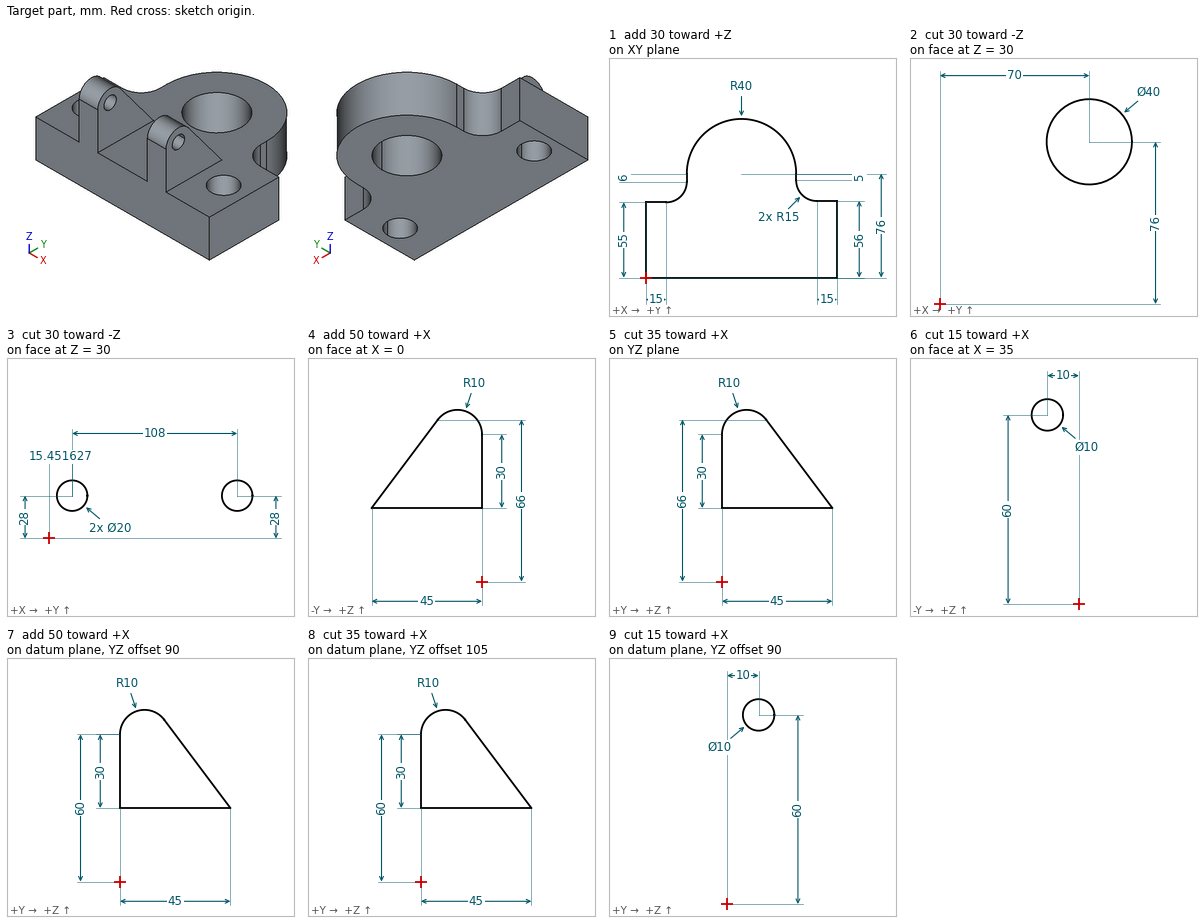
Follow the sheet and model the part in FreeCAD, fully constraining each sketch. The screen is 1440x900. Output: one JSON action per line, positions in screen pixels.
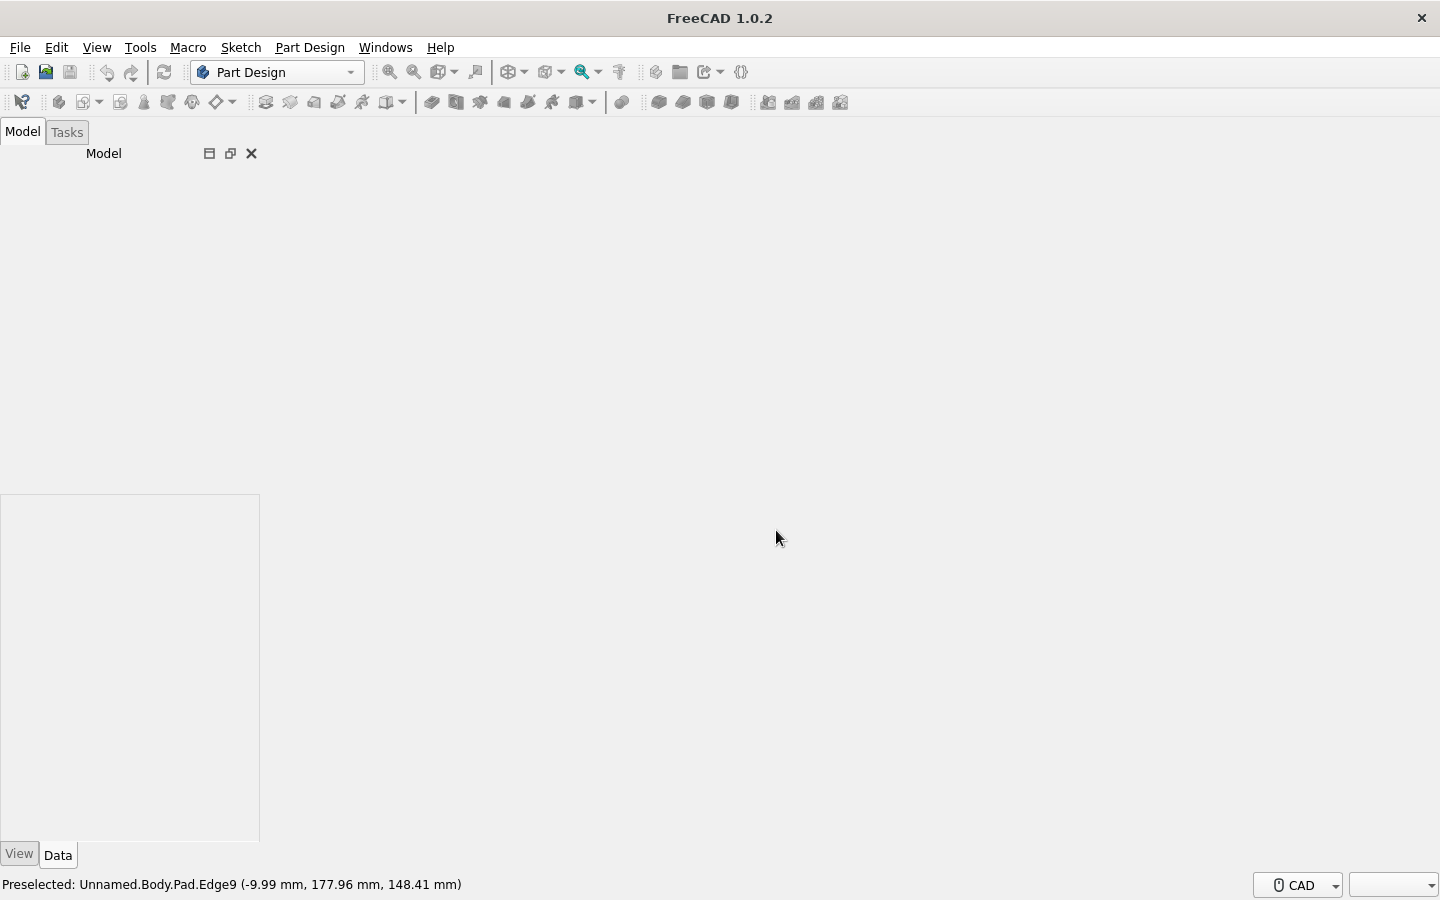
{"action": "key", "text": "ctrl+n"}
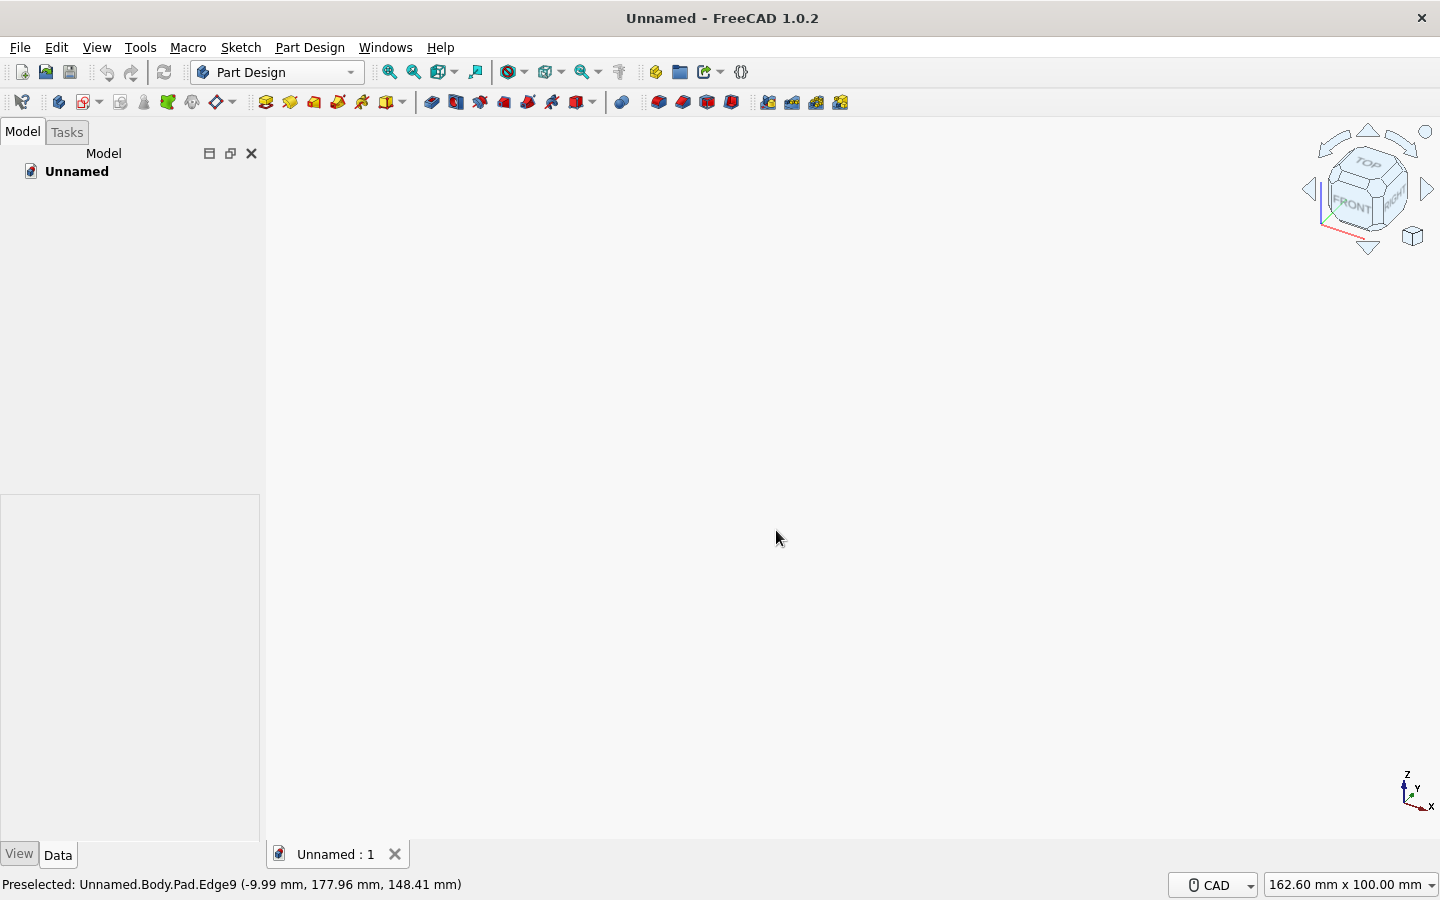
{"action": "left_click", "coordinate": [84, 102]}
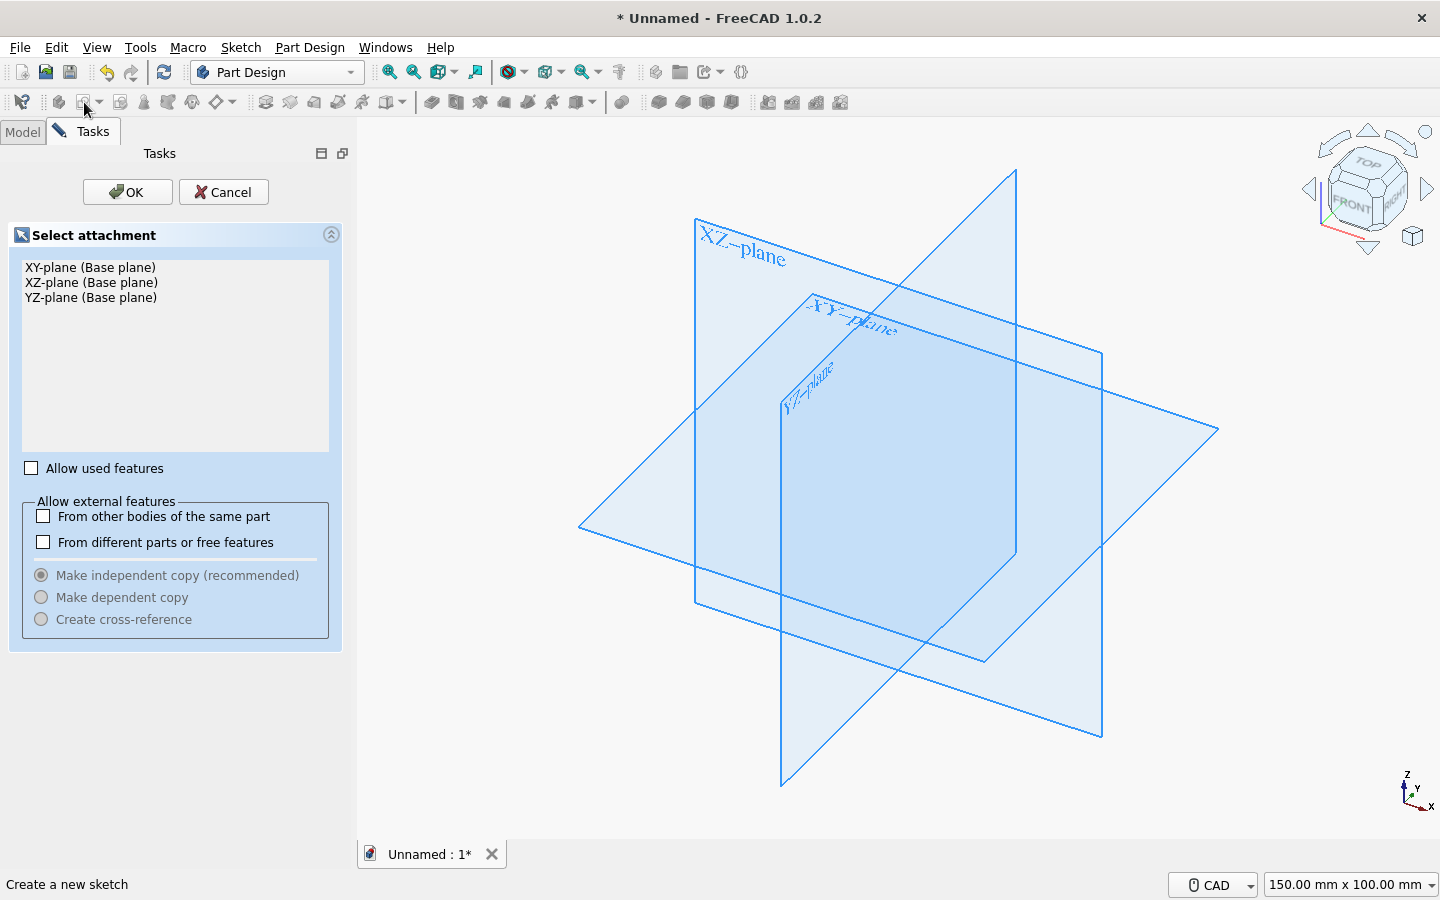
{"action": "left_click", "coordinate": [82, 268]}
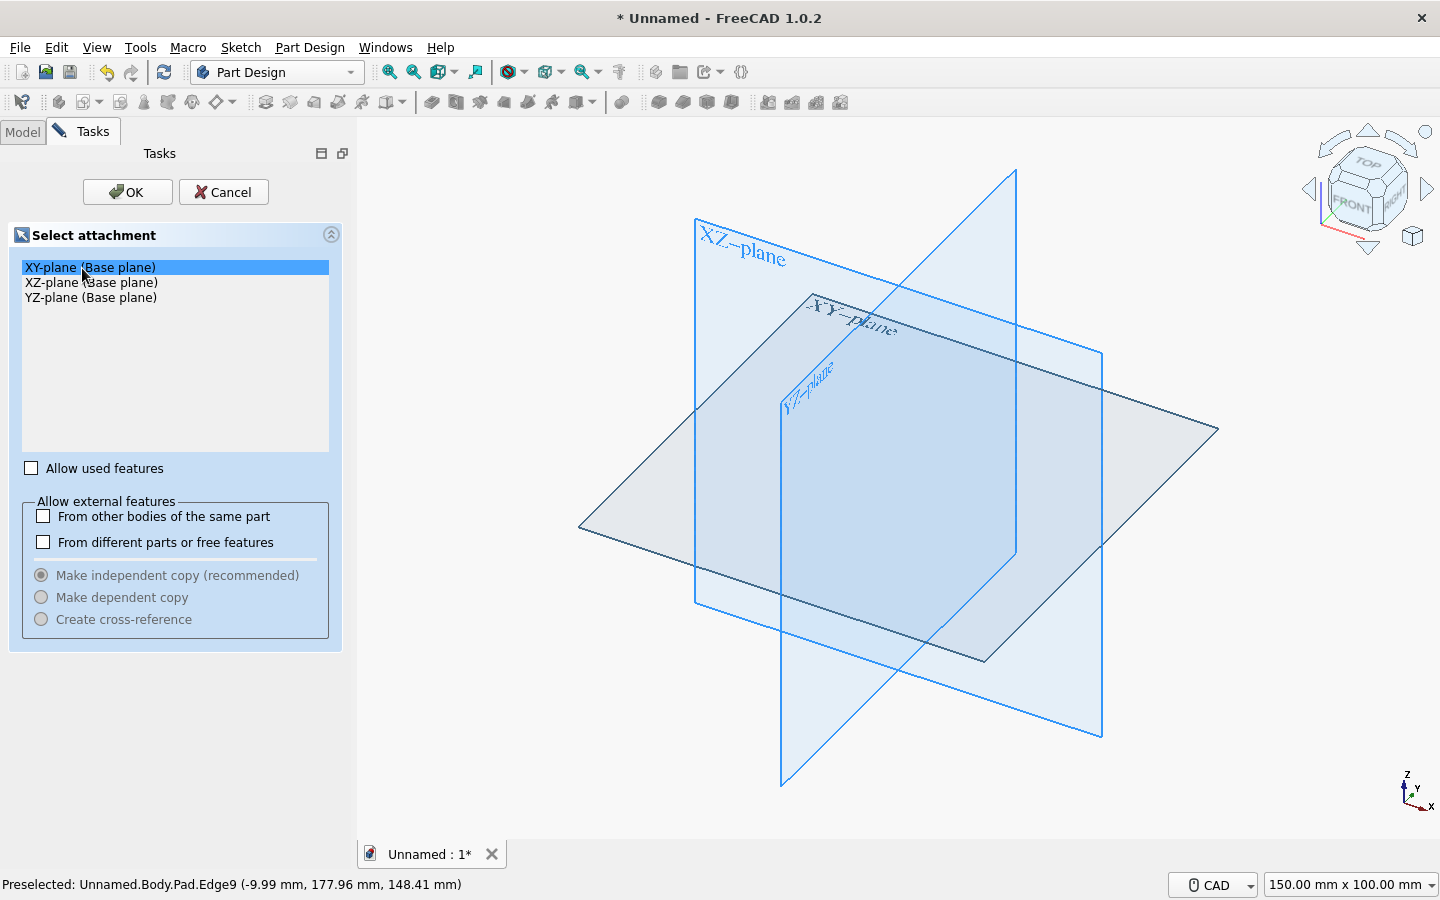
{"action": "left_click", "coordinate": [128, 192]}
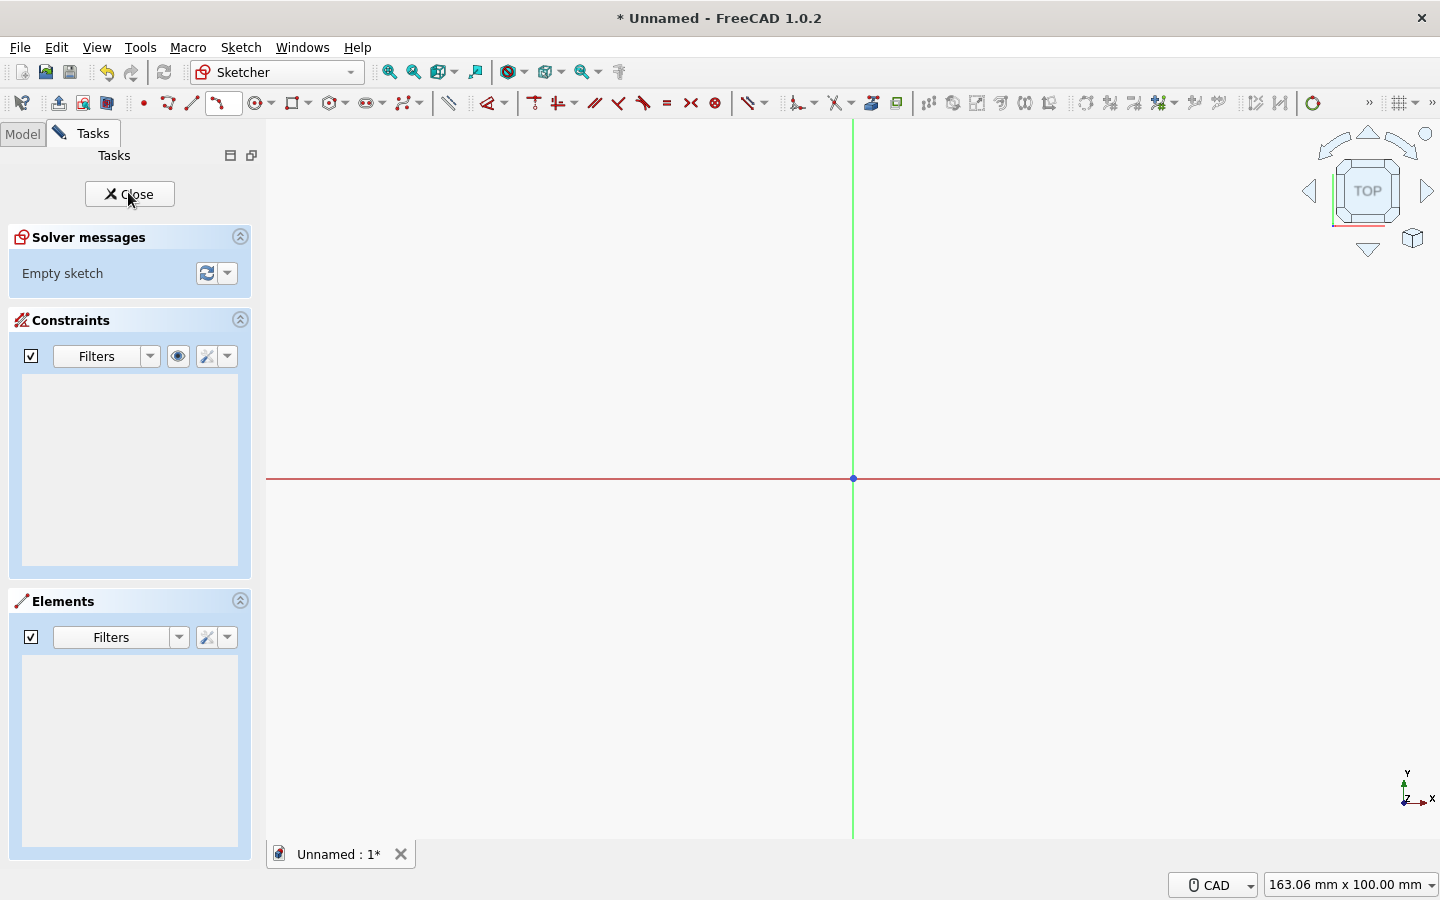
{"action": "scroll", "coordinate": [317, 811], "scroll_direction": "down", "scroll_amount": 4}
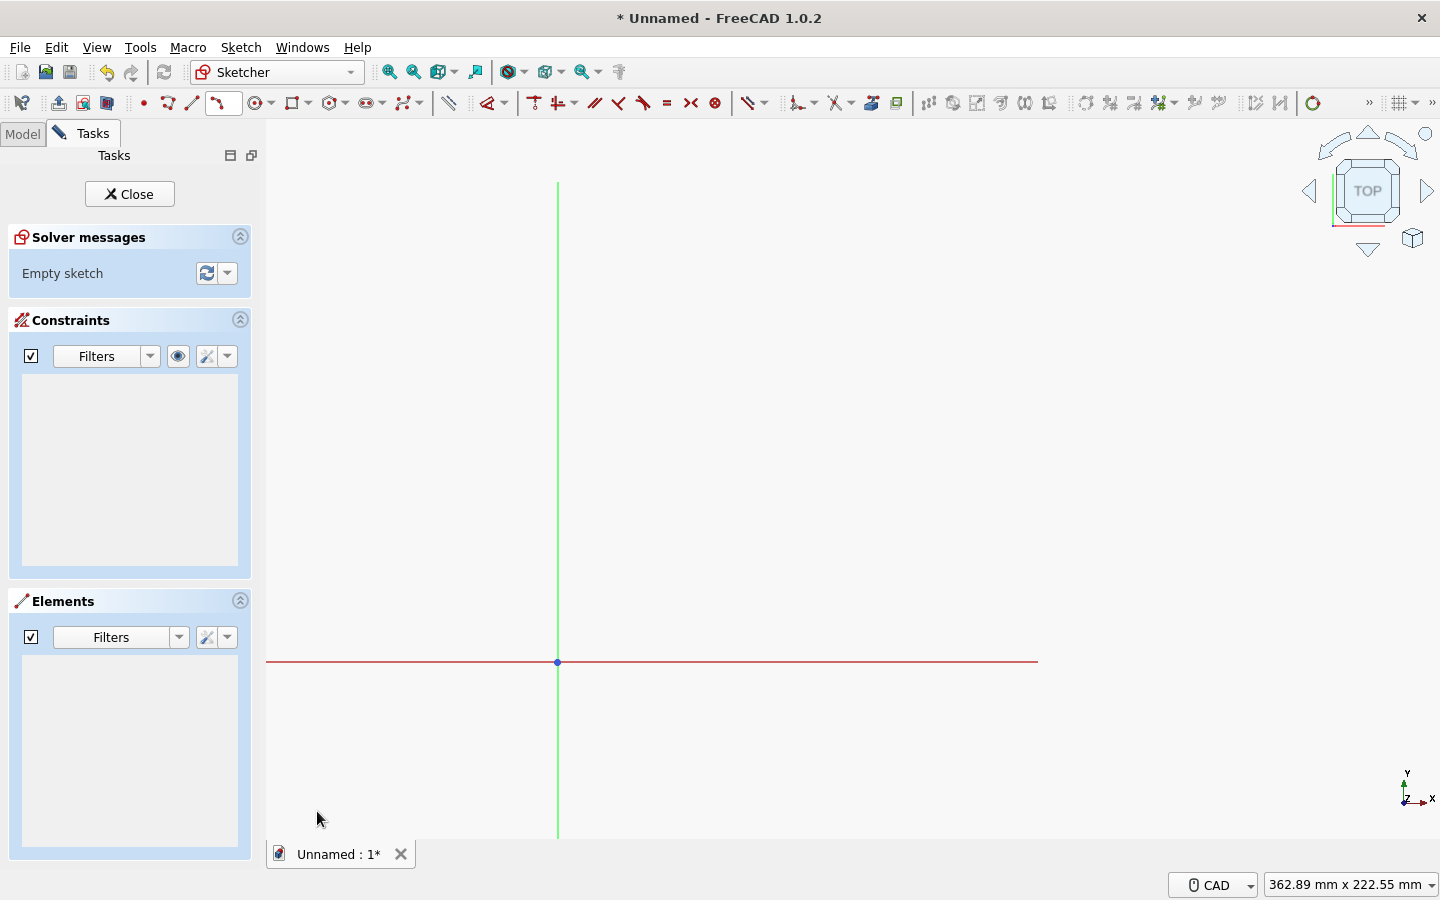
{"action": "key", "text": "g l"}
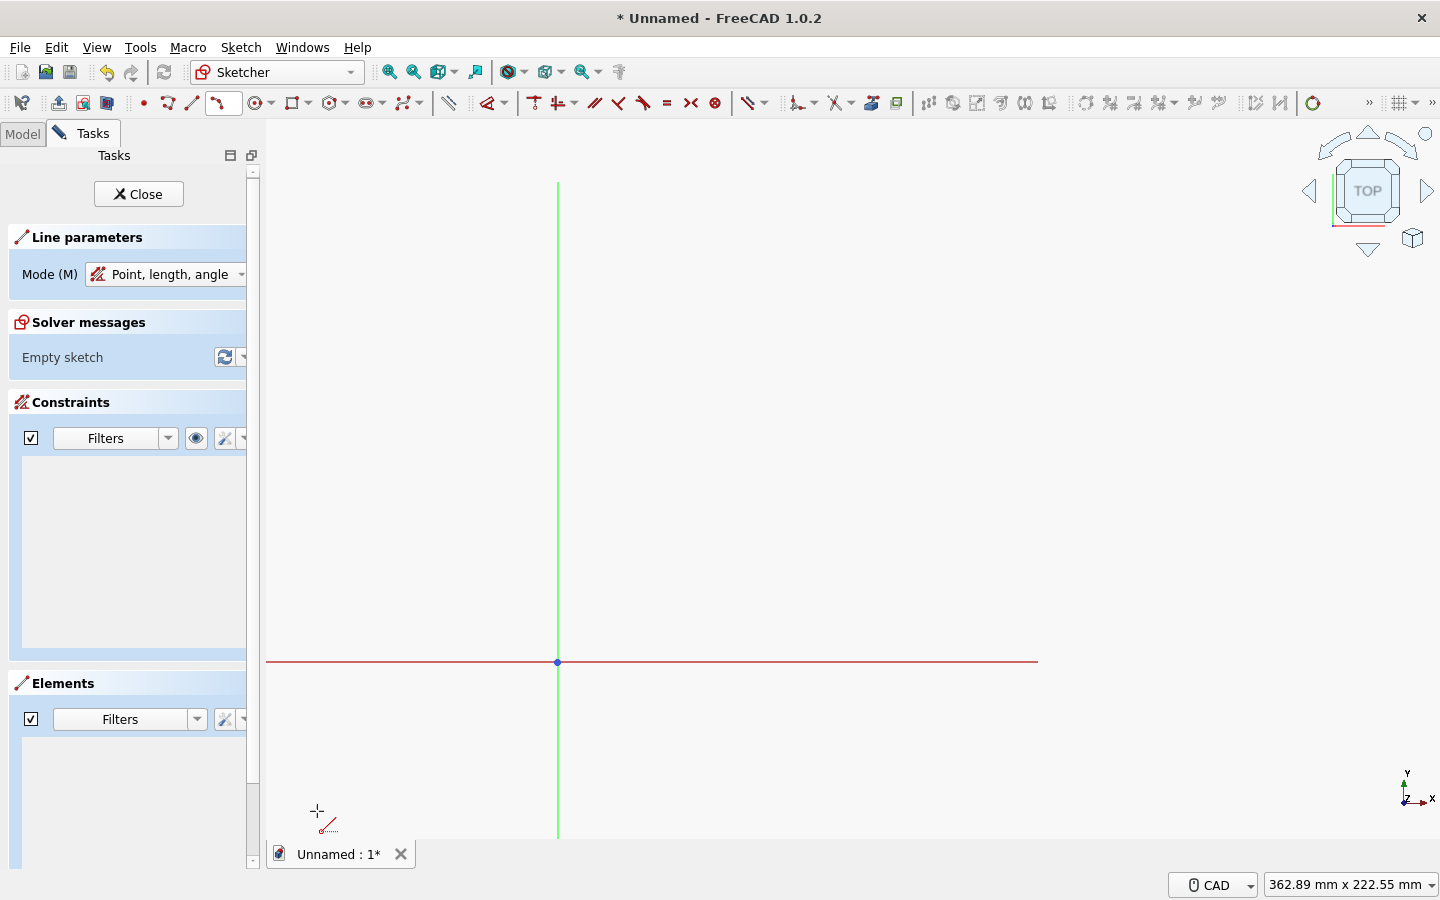
{"action": "left_click", "coordinate": [914, 433]}
{"action": "left_click", "coordinate": [914, 416]}